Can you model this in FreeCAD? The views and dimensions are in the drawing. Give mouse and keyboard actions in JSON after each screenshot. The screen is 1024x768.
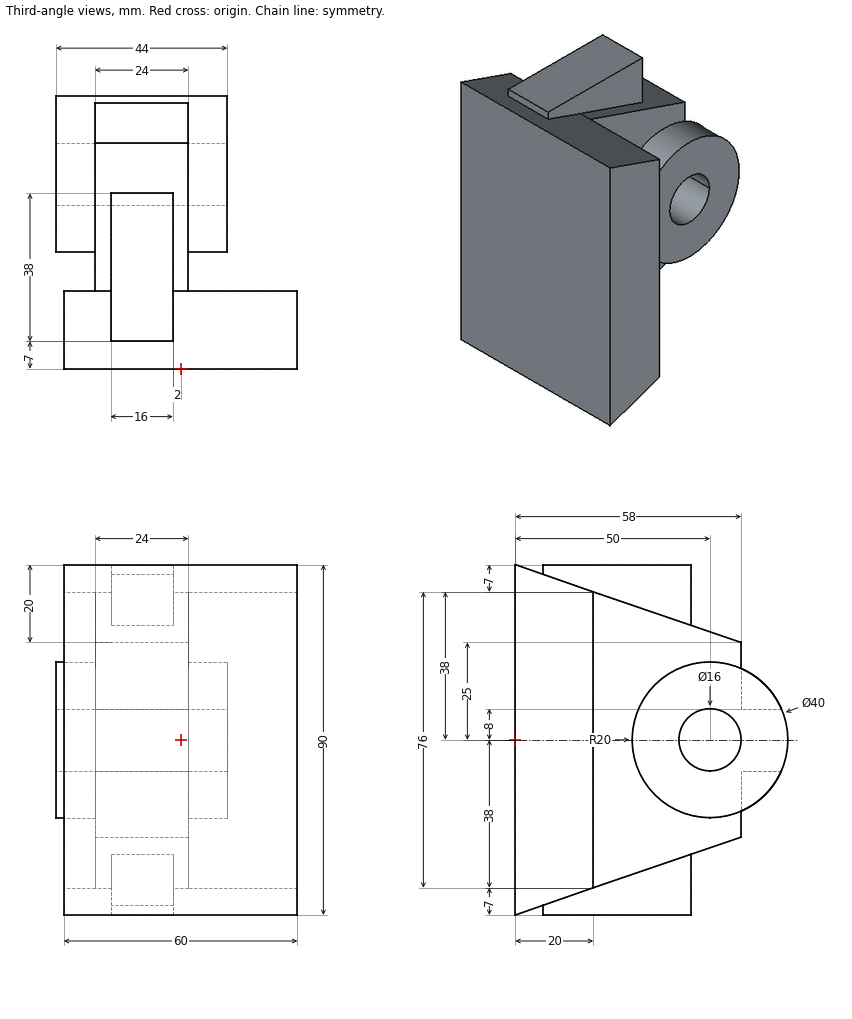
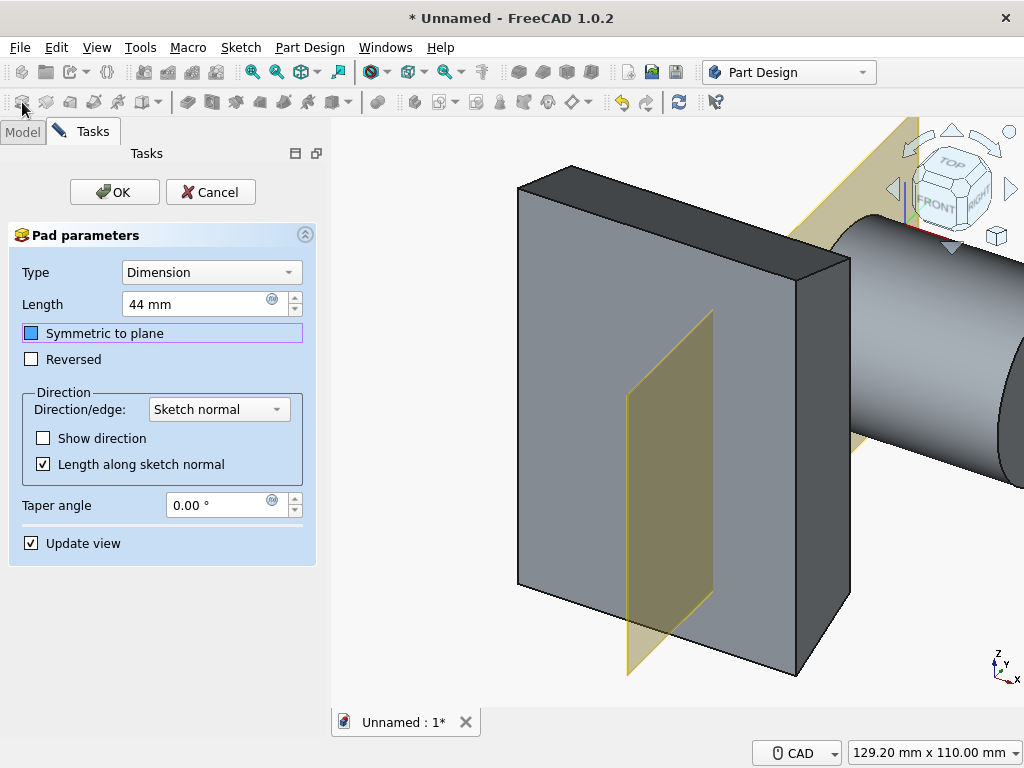
{"action": "left_click", "coordinate": [30, 359]}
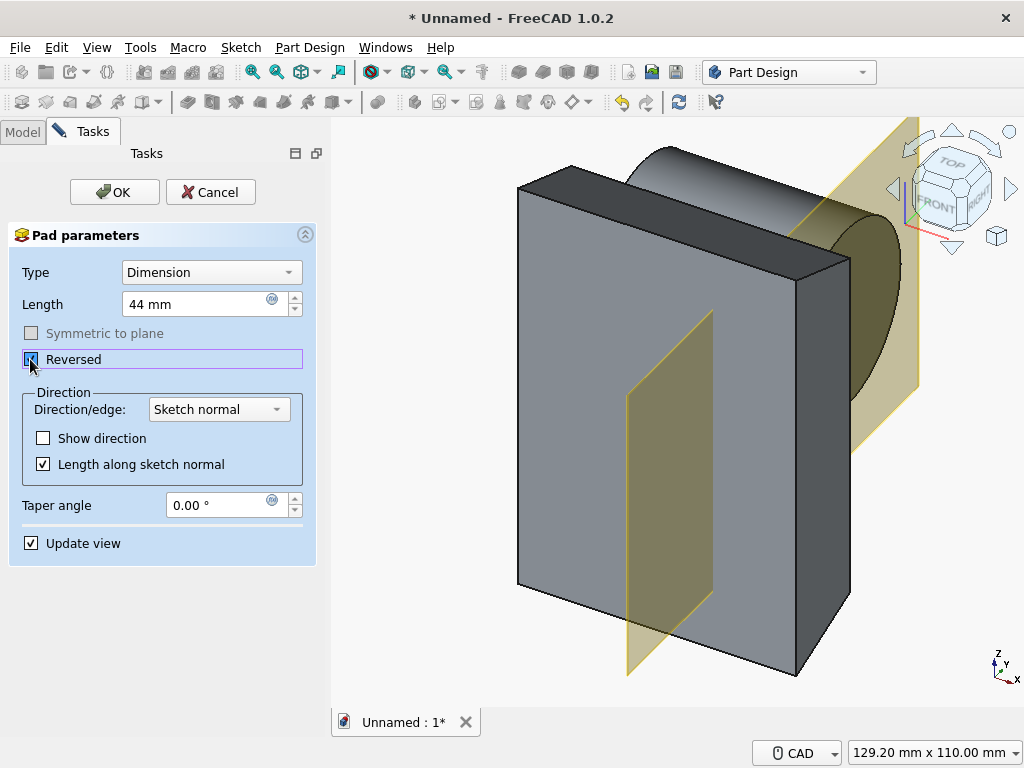
{"action": "left_click", "coordinate": [115, 192]}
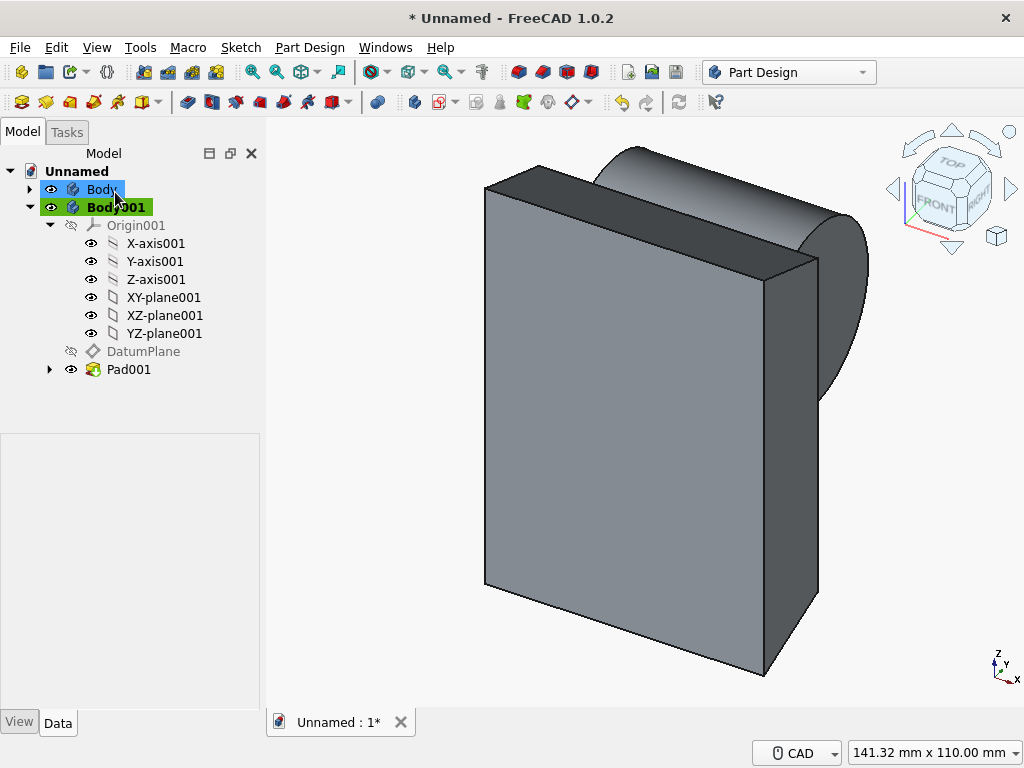
{"action": "left_click", "coordinate": [254, 72]}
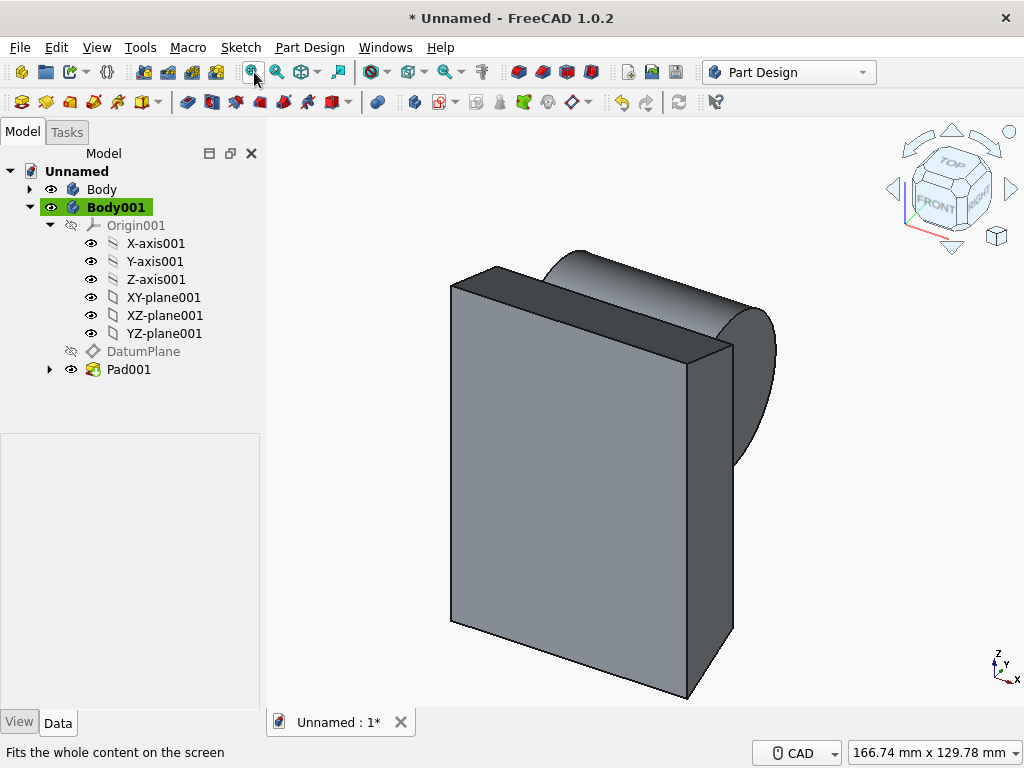
{"action": "double_click", "coordinate": [96, 189]}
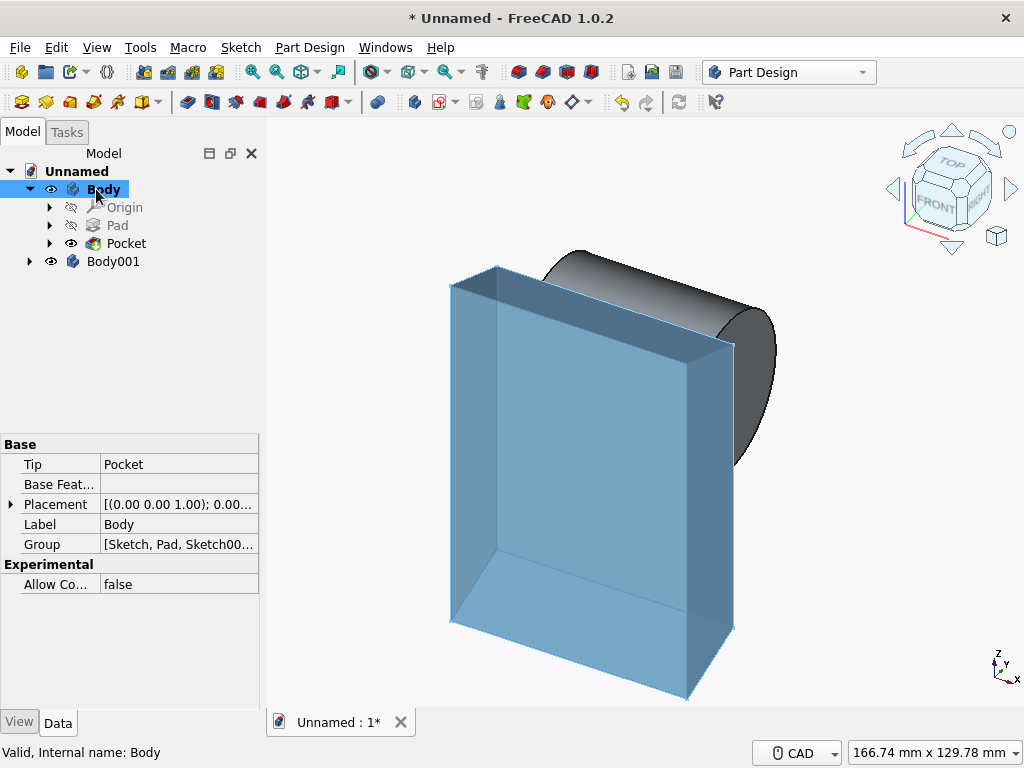
{"action": "left_click", "coordinate": [96, 189]}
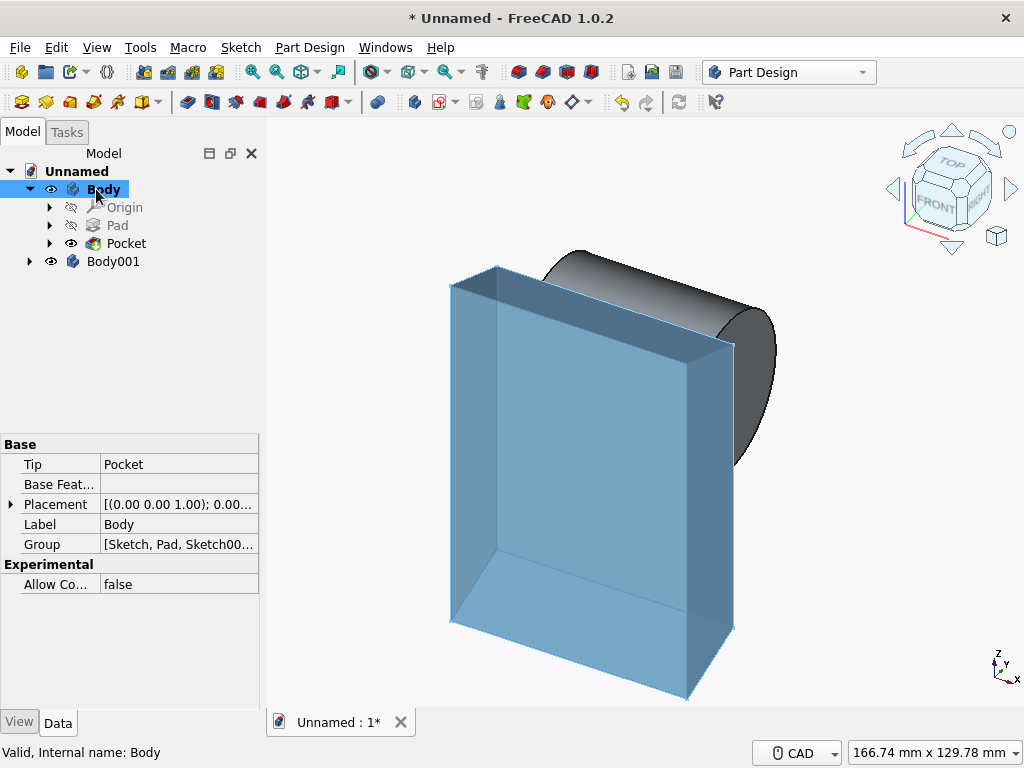
{"action": "left_click", "coordinate": [146, 584]}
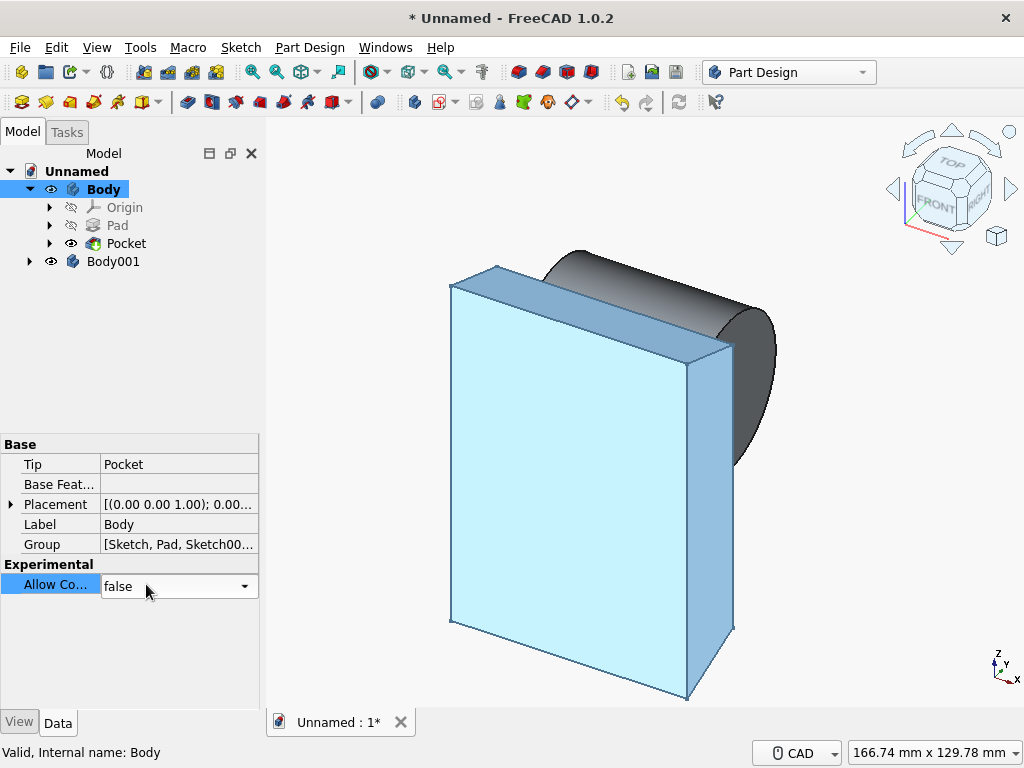
{"action": "left_click", "coordinate": [146, 584]}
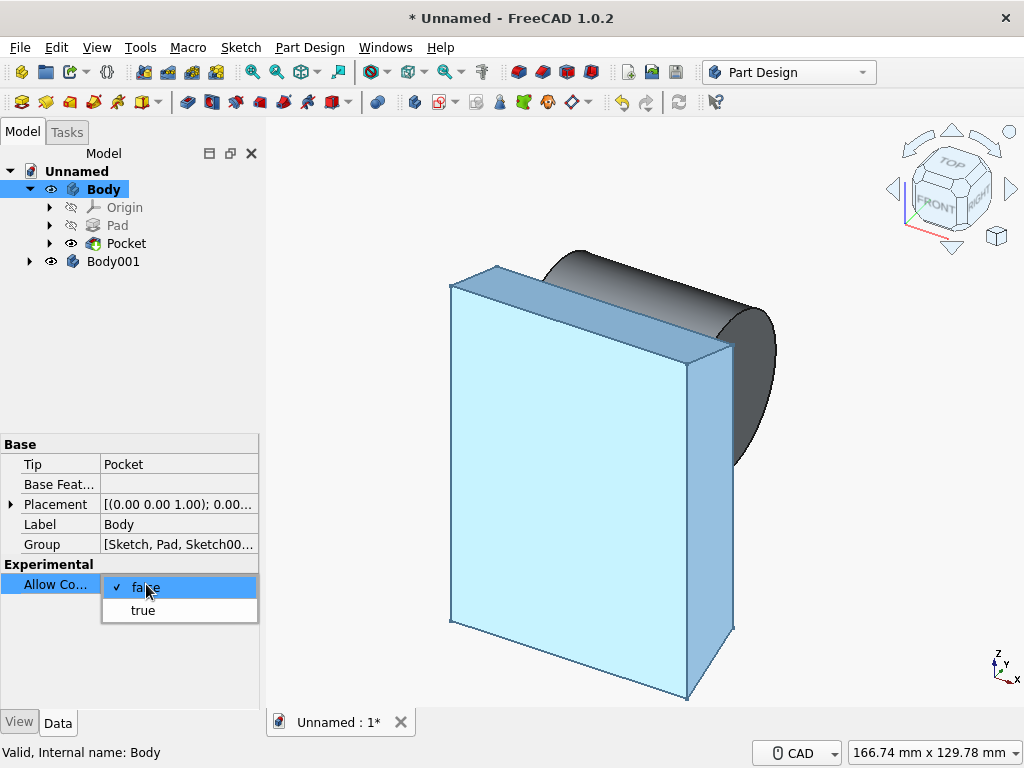
{"action": "left_click", "coordinate": [179, 610]}
{"action": "key", "text": "Return"}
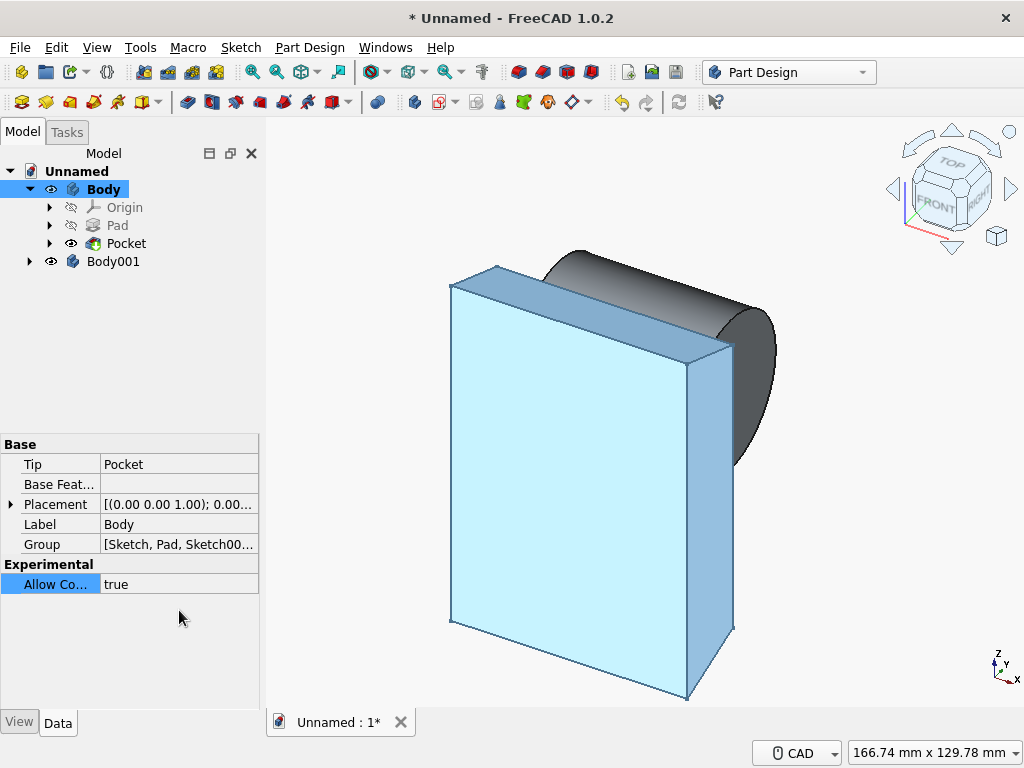
{"action": "left_click", "coordinate": [96, 261]}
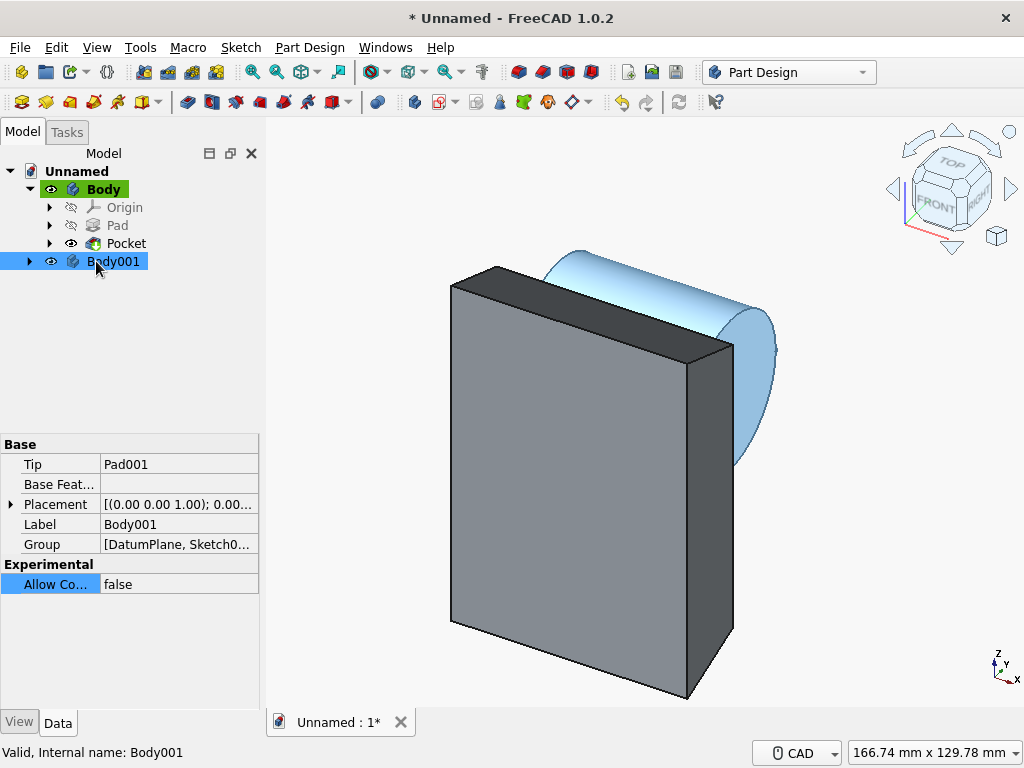
{"action": "left_click", "coordinate": [378, 102]}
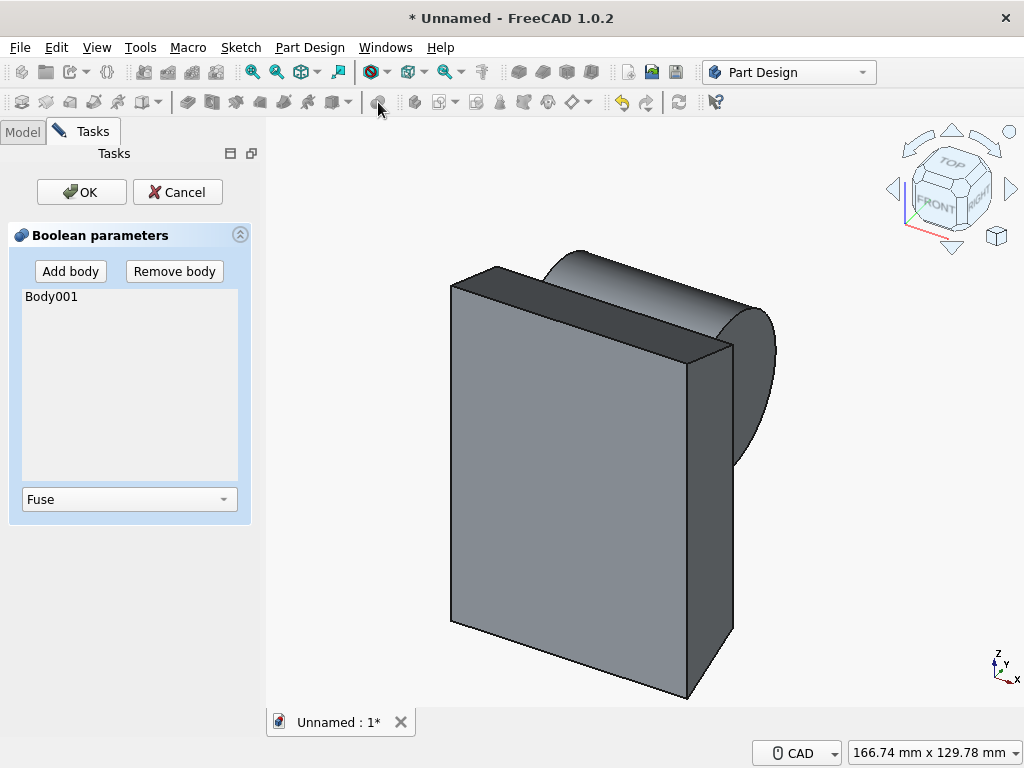
{"action": "left_click", "coordinate": [82, 192]}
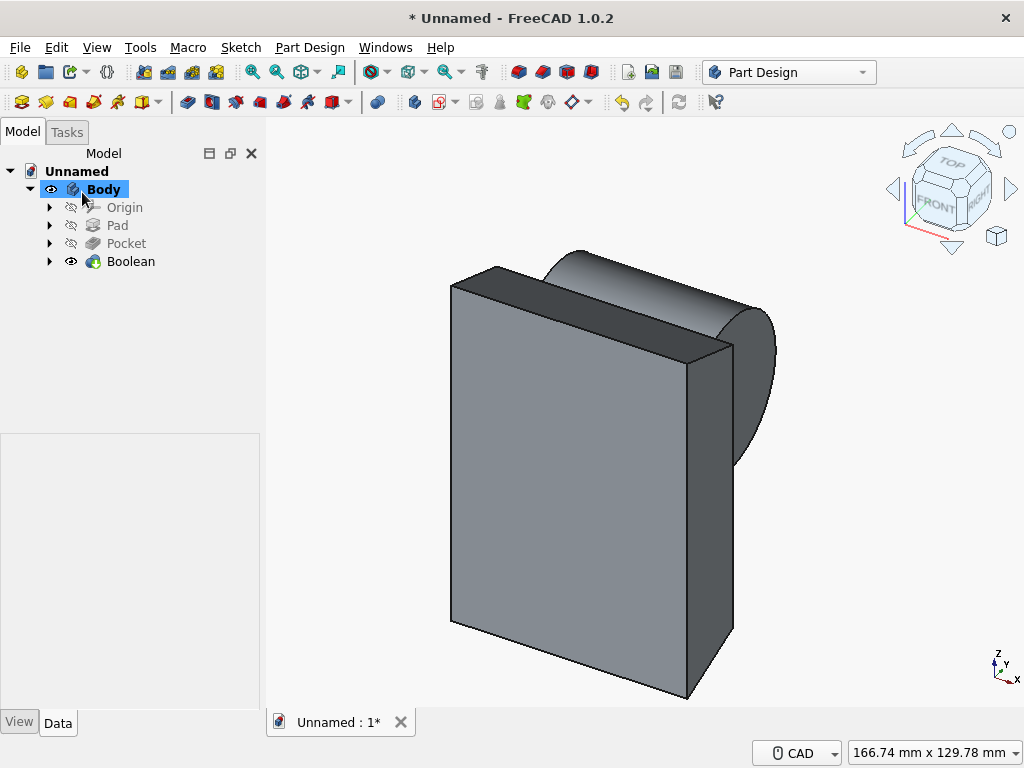
{"action": "left_click", "coordinate": [50, 207]}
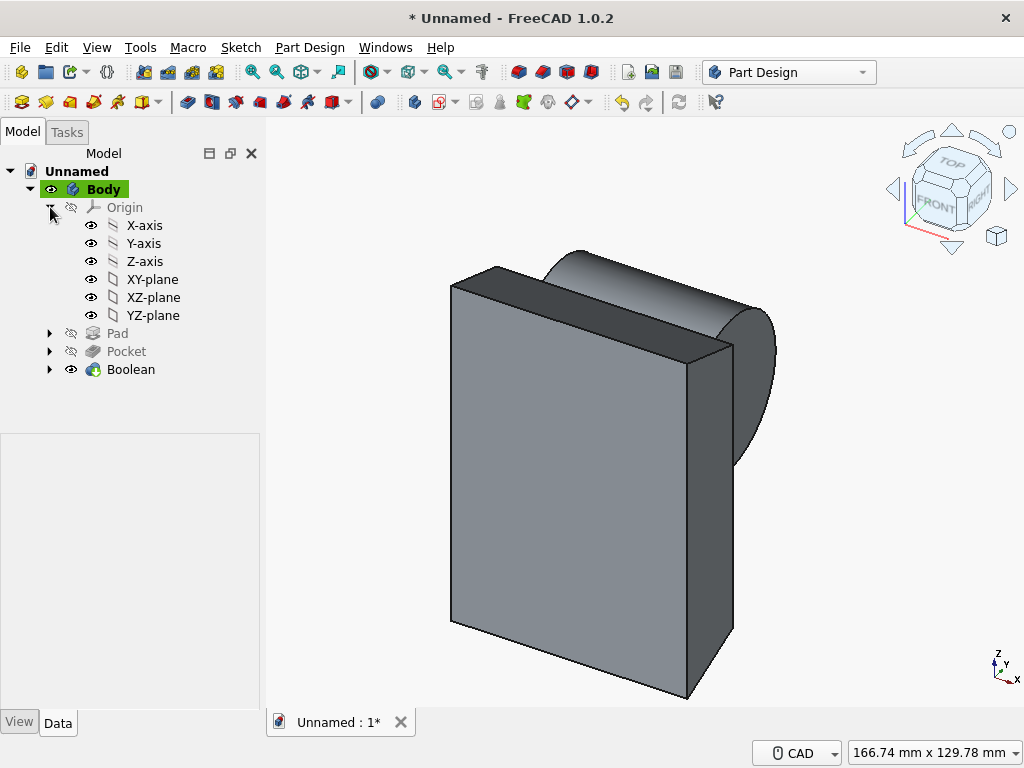
{"action": "left_click", "coordinate": [136, 315]}